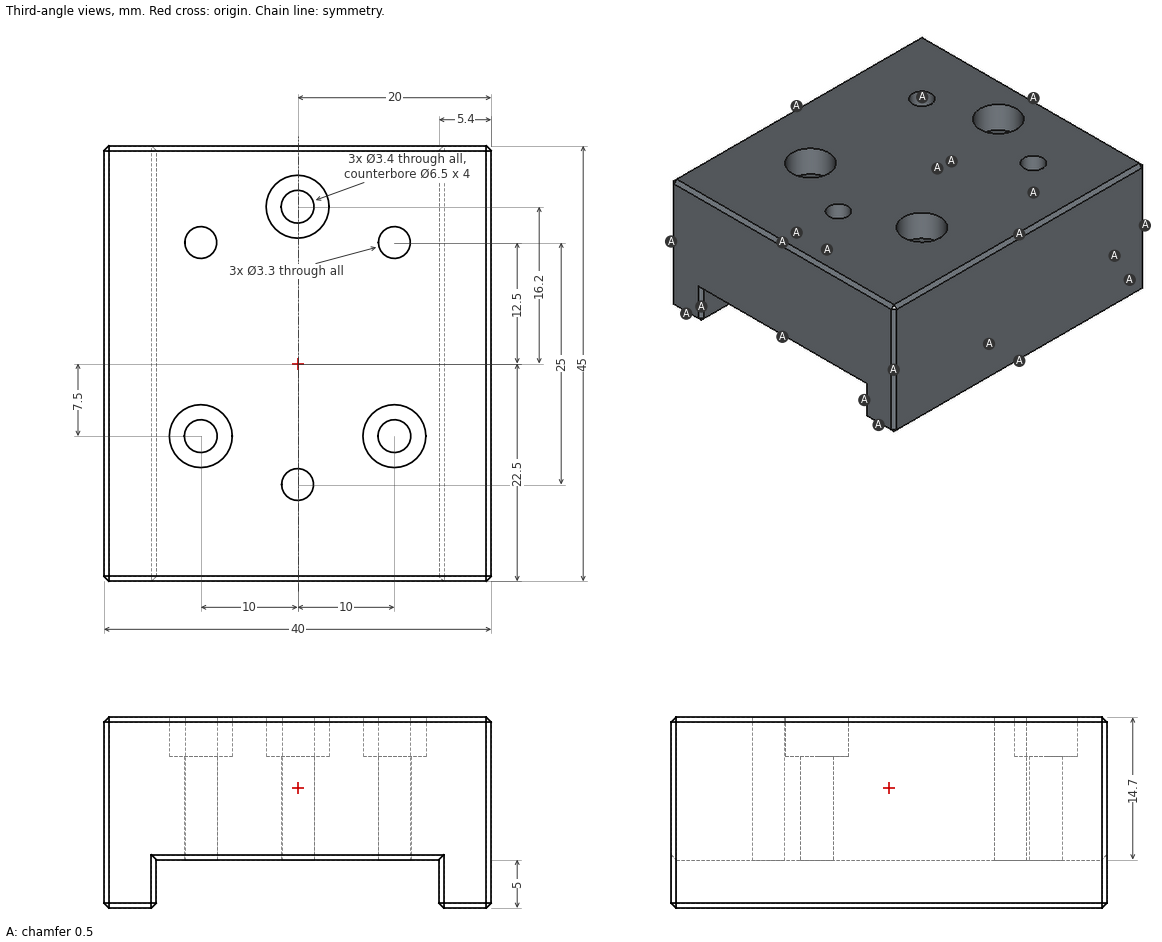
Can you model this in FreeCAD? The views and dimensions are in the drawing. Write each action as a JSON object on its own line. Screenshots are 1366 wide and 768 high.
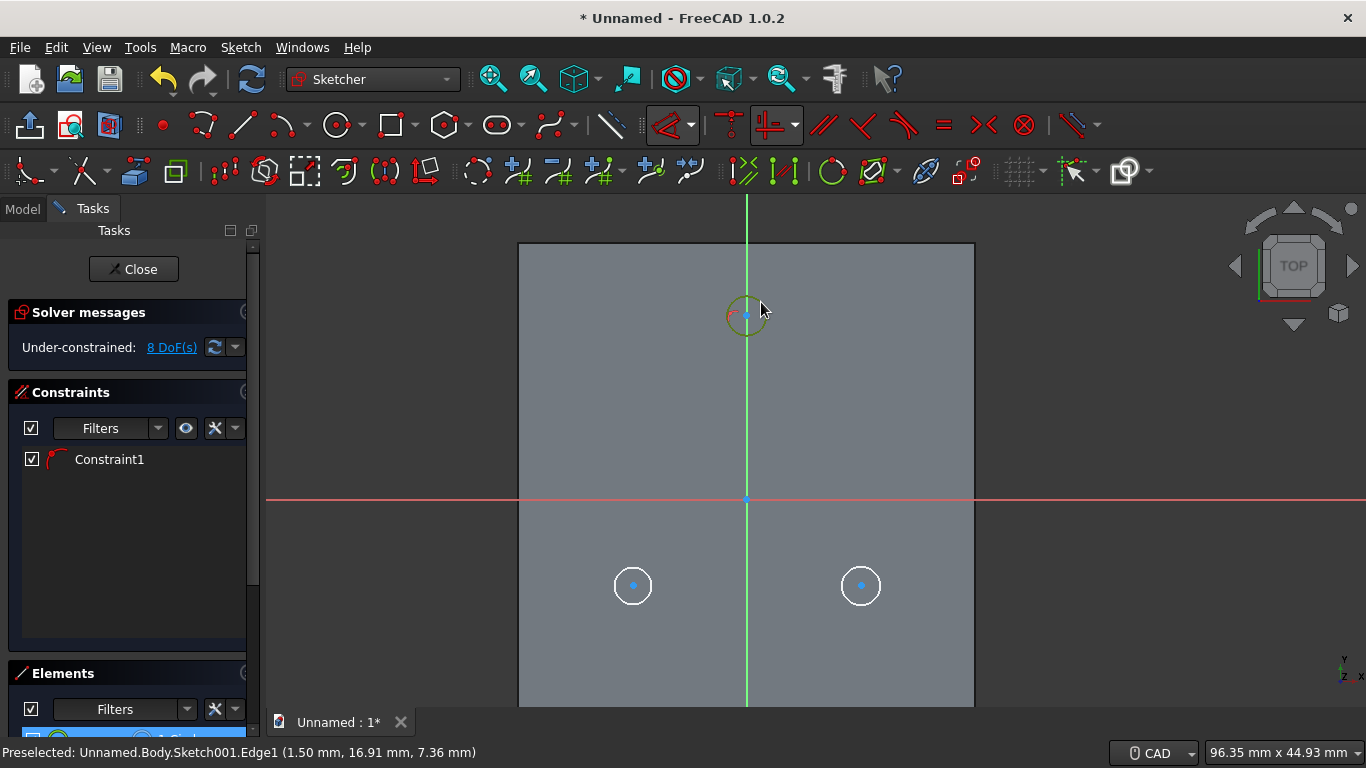
{"action": "left_click", "coordinate": [646, 573]}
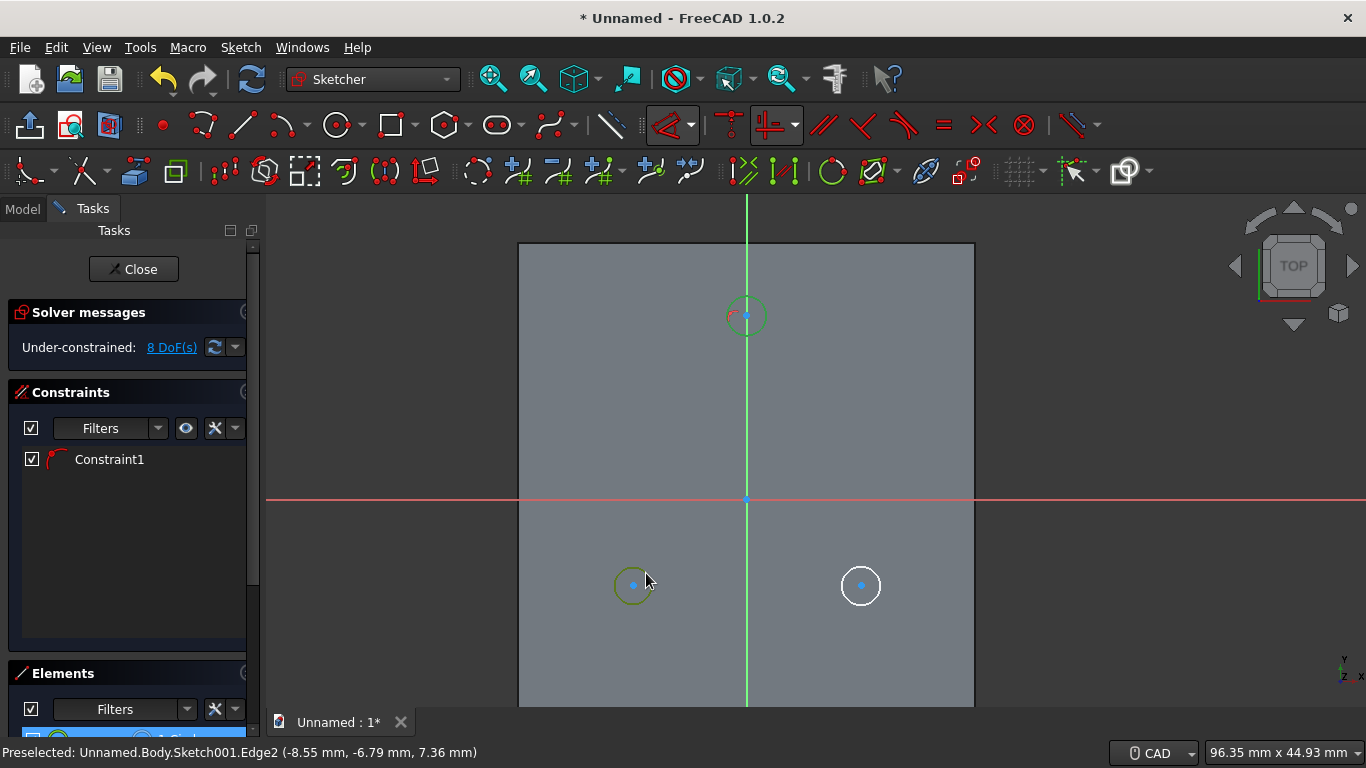
{"action": "left_click", "coordinate": [874, 572]}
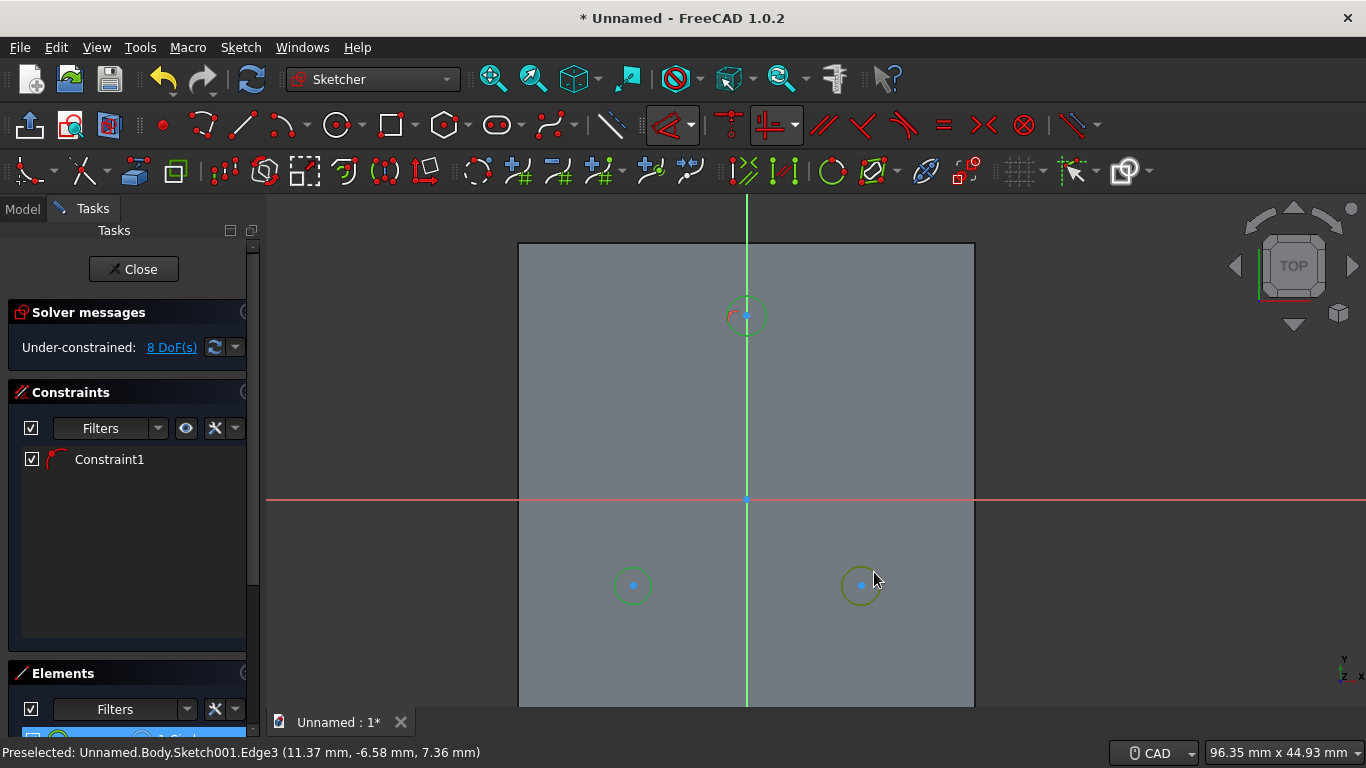
{"action": "left_click", "coordinate": [944, 126]}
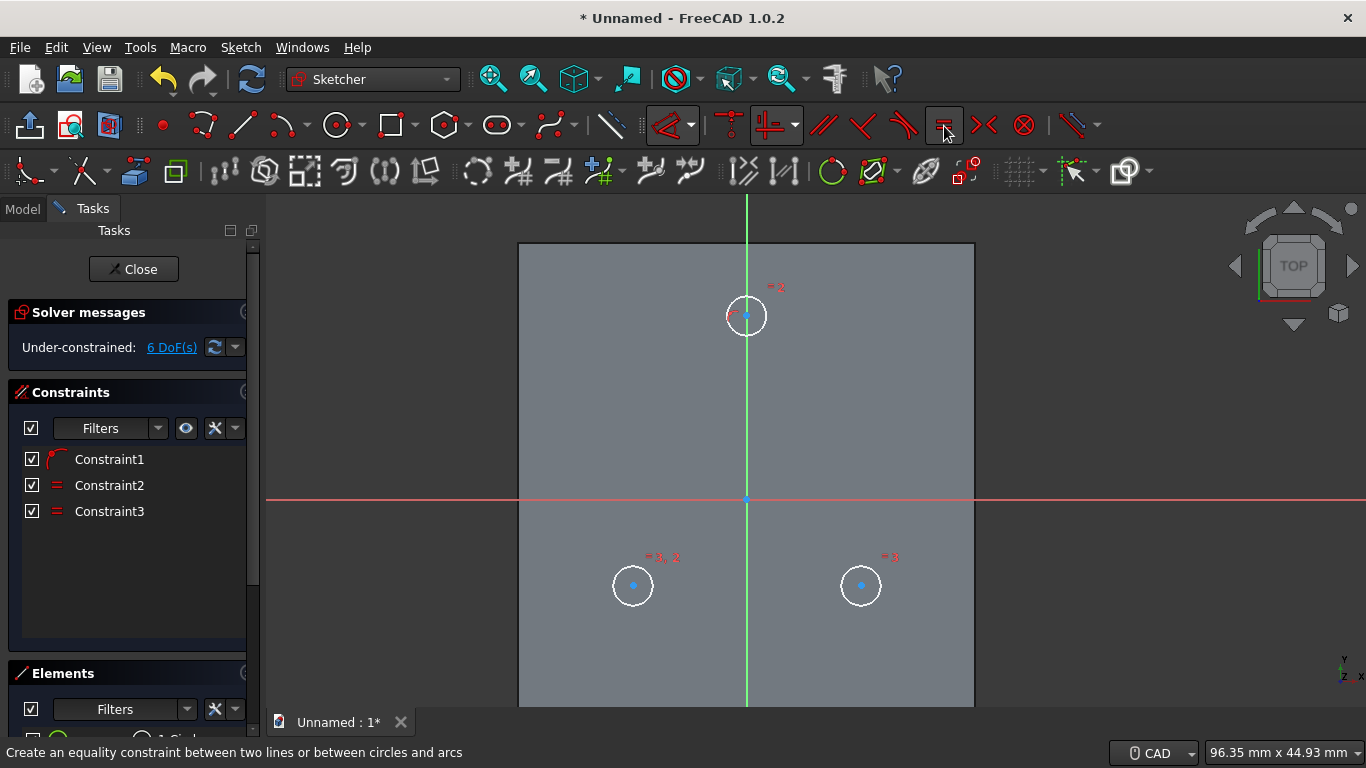
{"action": "left_click", "coordinate": [633, 586]}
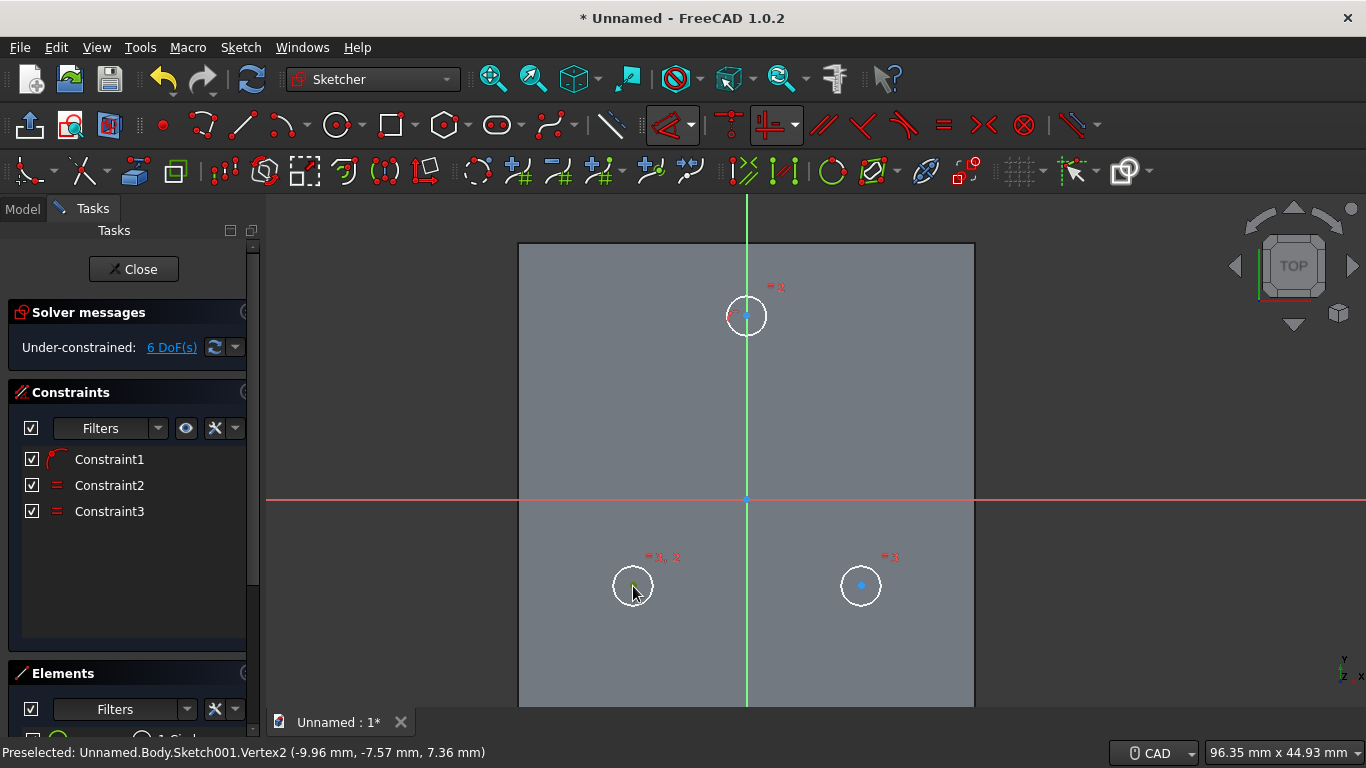
{"action": "left_click", "coordinate": [861, 586]}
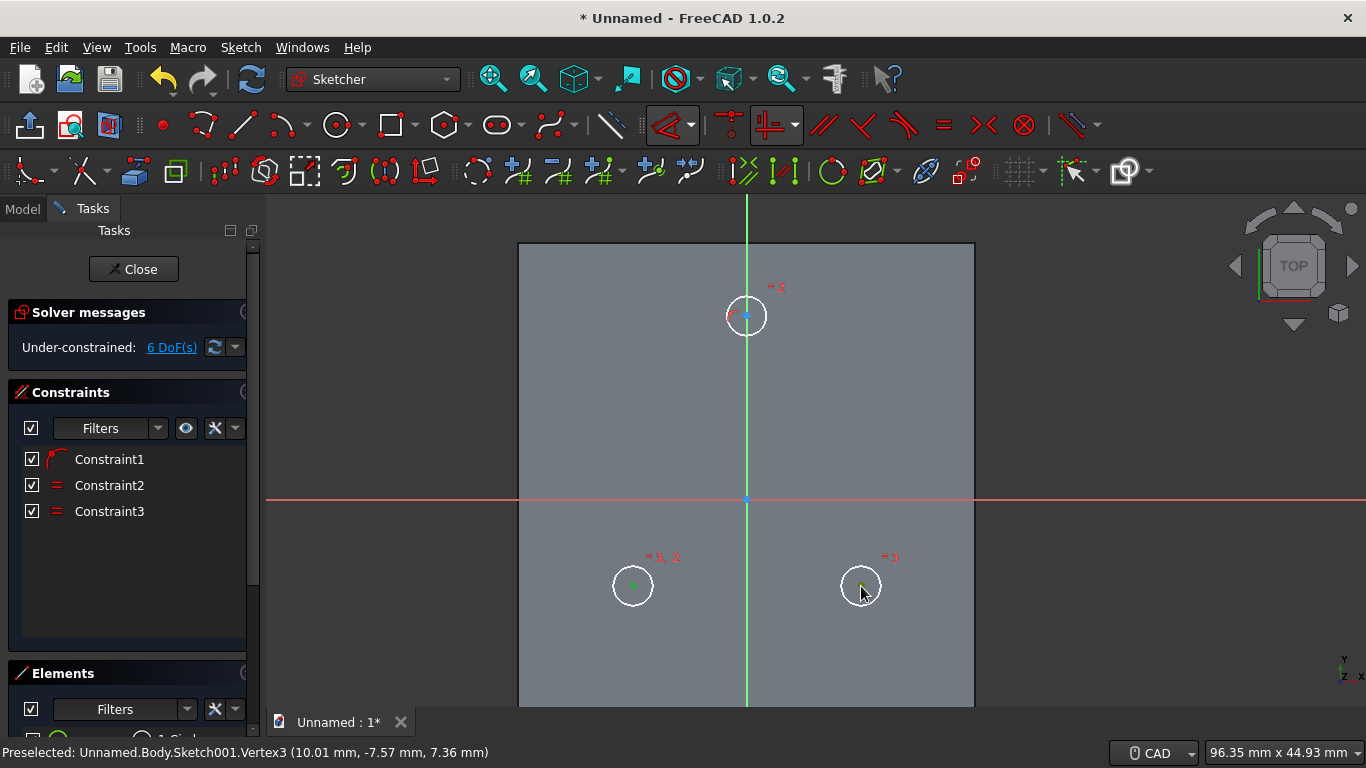
{"action": "left_click", "coordinate": [798, 126]}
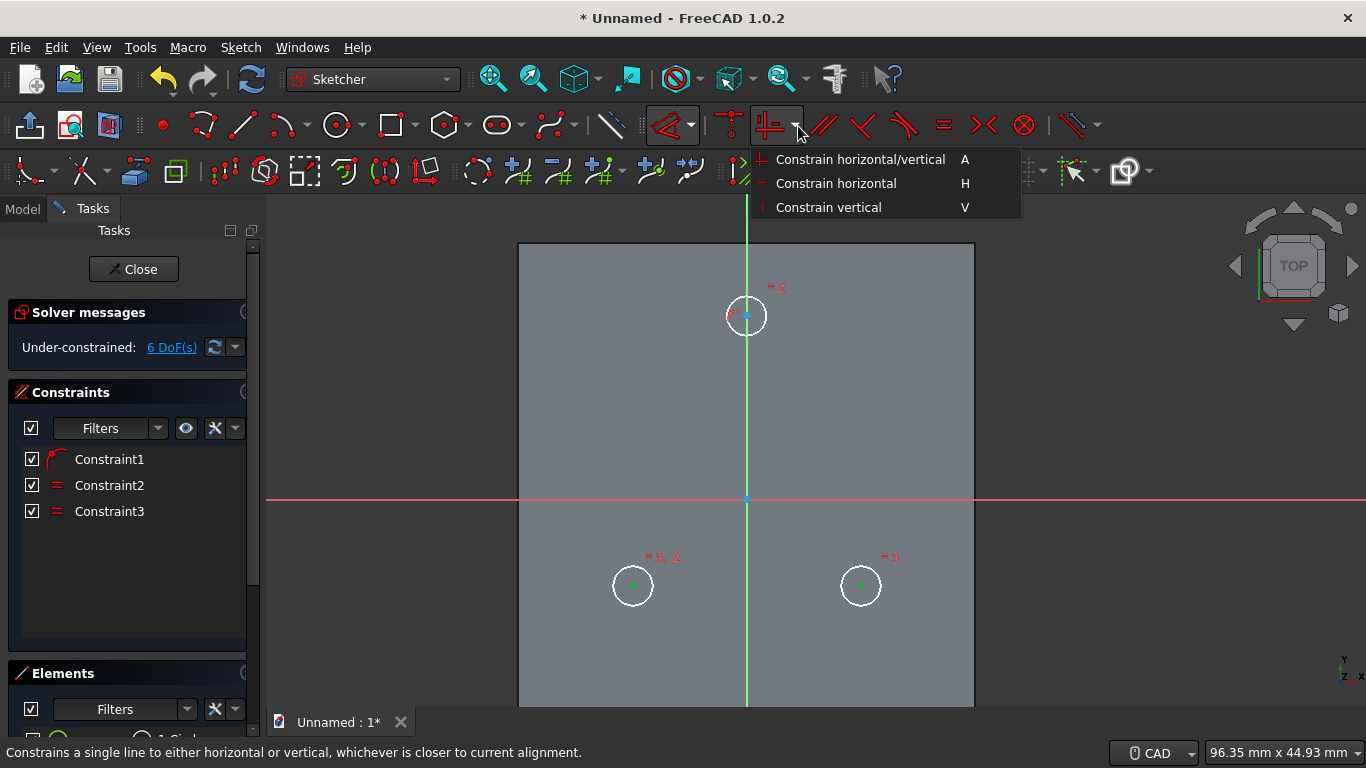
{"action": "left_click", "coordinate": [886, 183]}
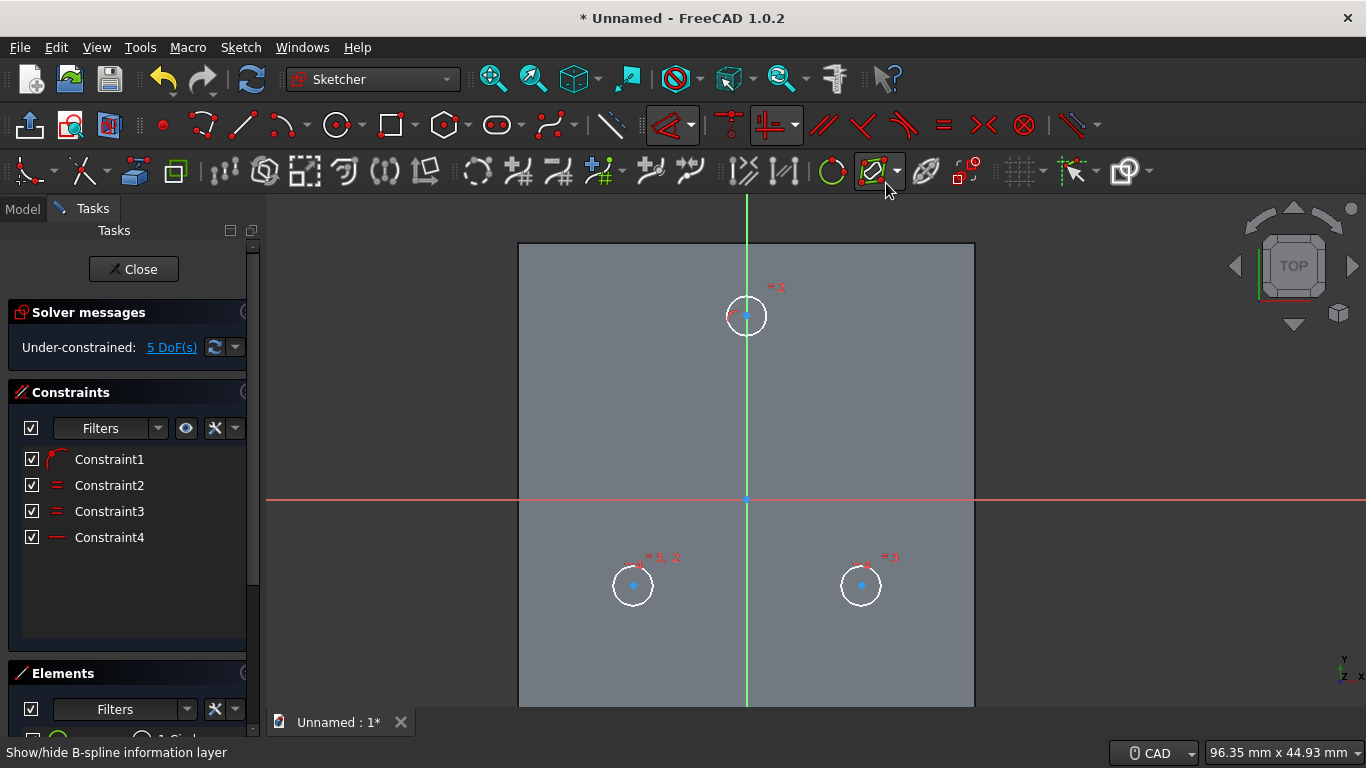
{"action": "left_click", "coordinate": [761, 302]}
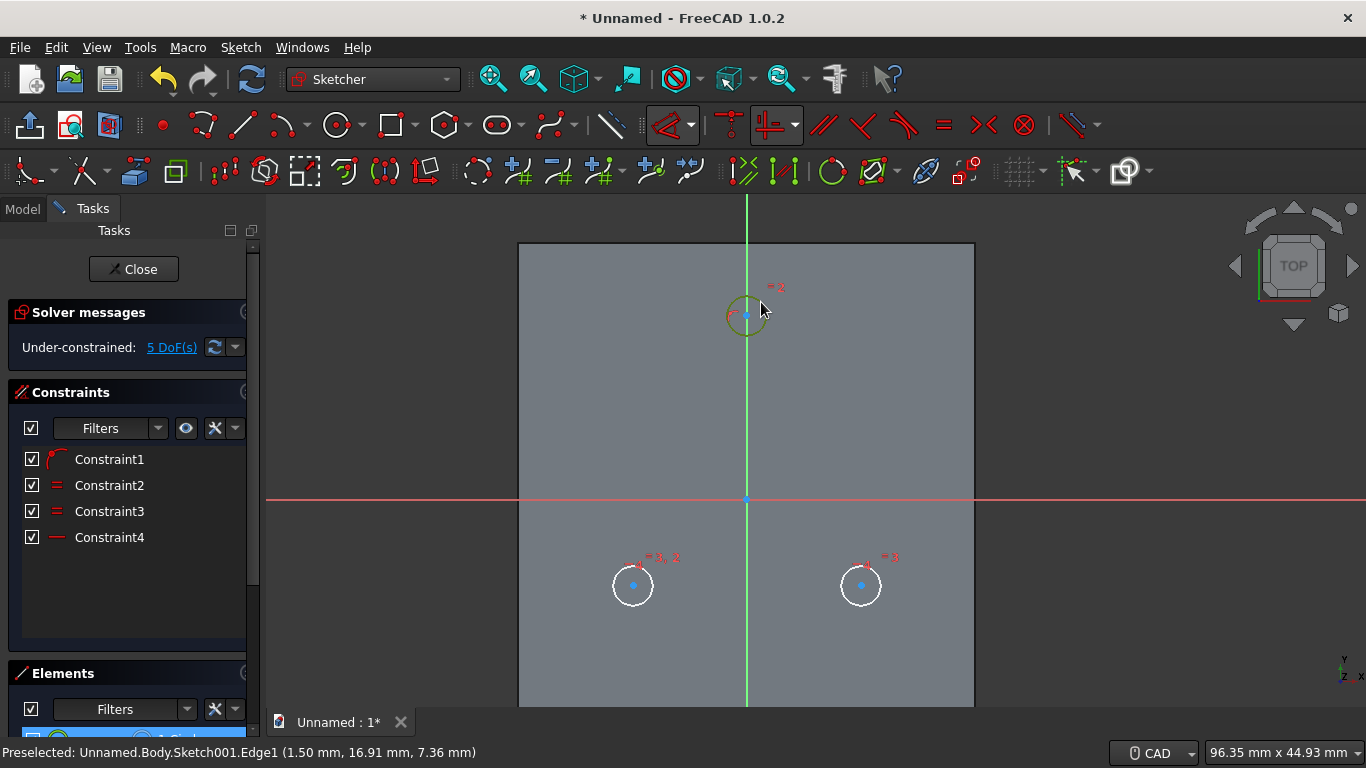
{"action": "key", "text": "k o"}